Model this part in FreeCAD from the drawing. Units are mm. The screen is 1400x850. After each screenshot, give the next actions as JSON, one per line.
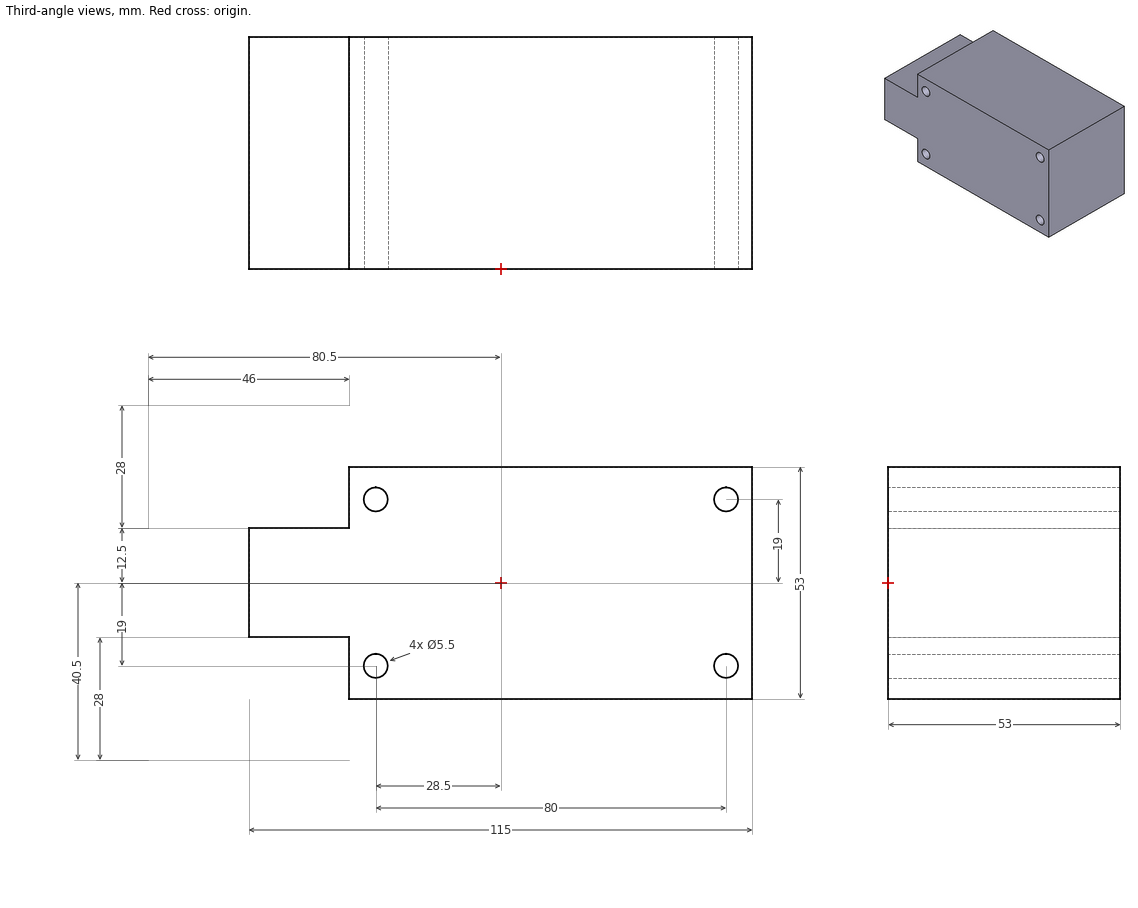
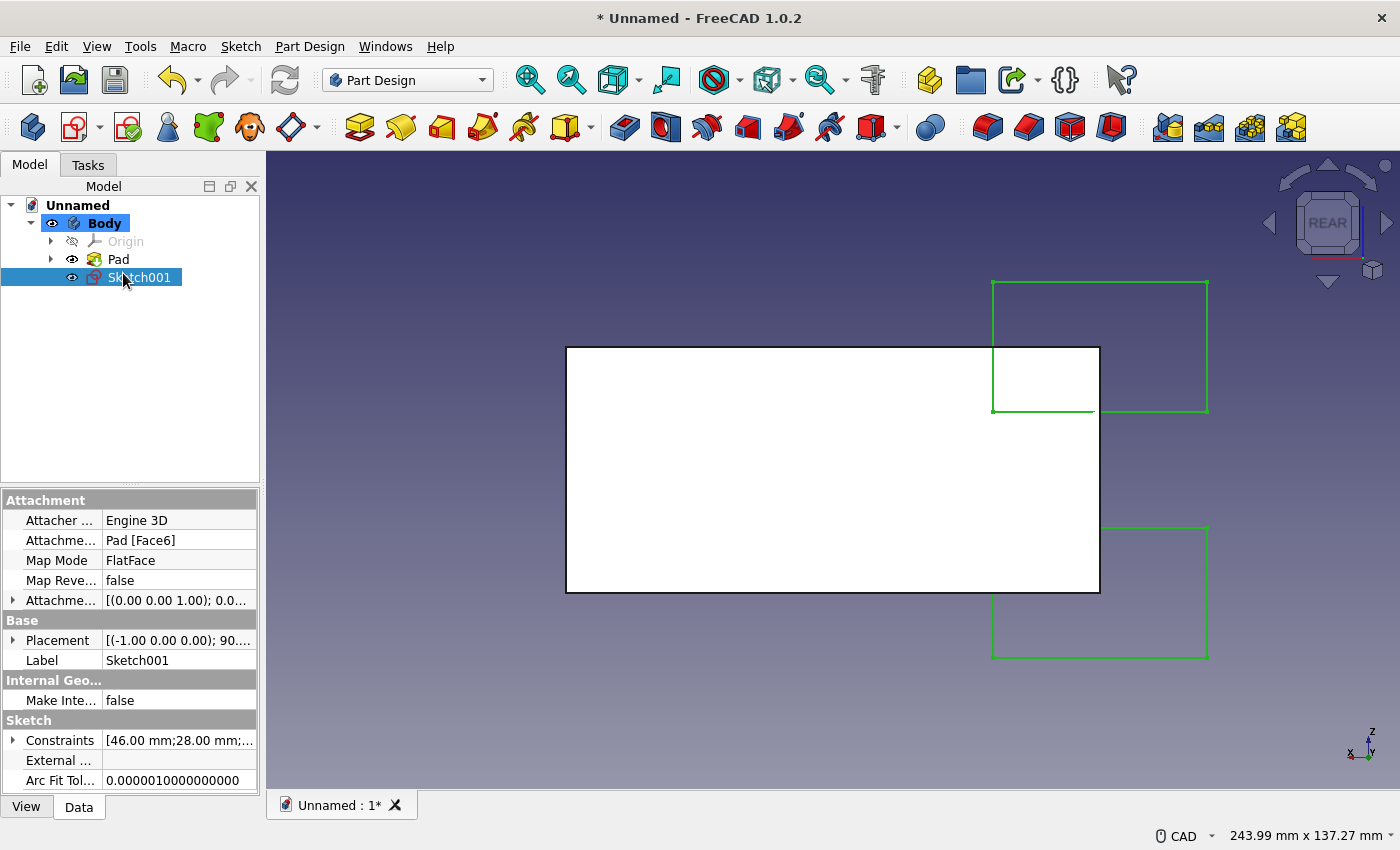
{"action": "left_click", "coordinate": [625, 128]}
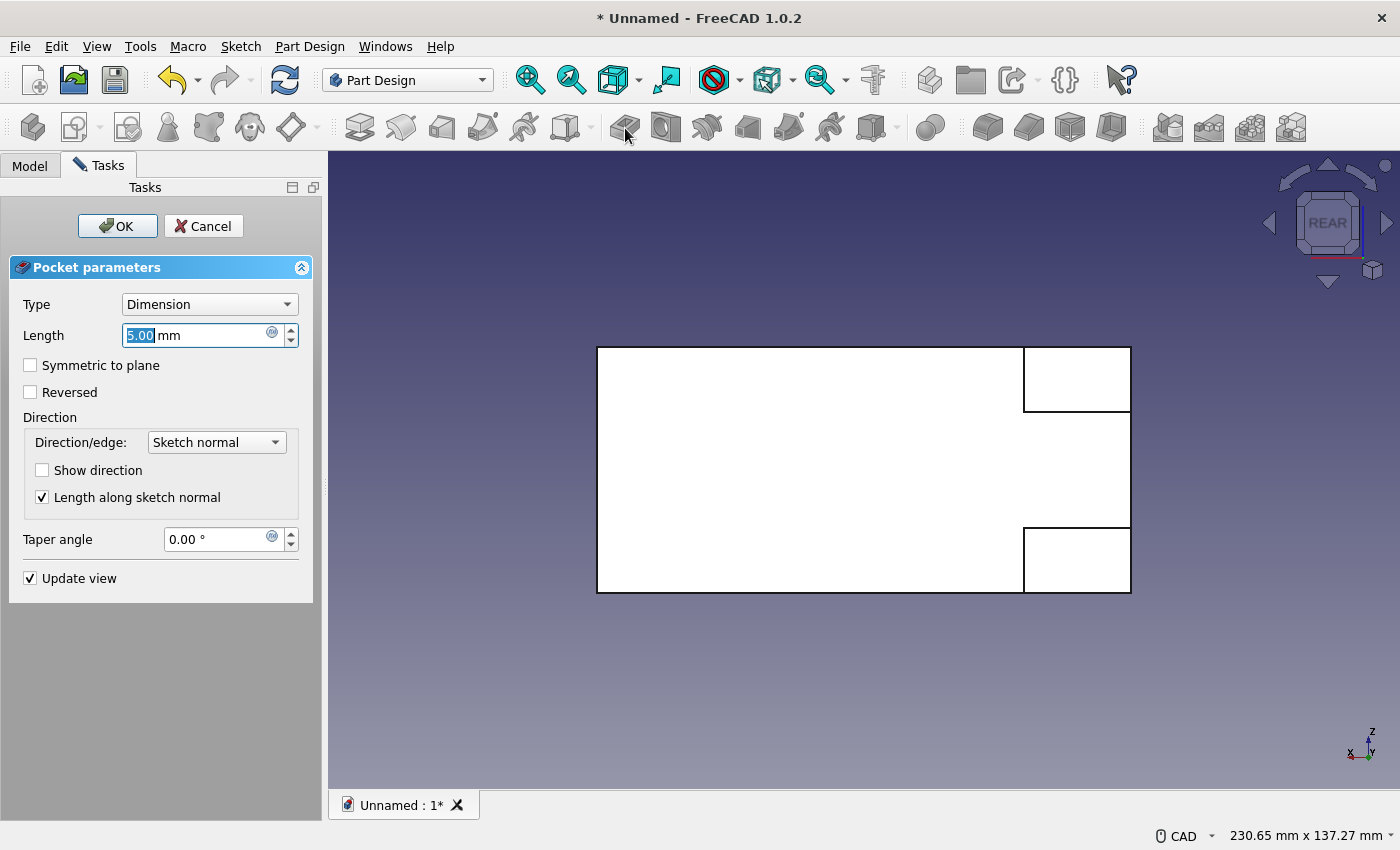
{"action": "left_click", "coordinate": [210, 304]}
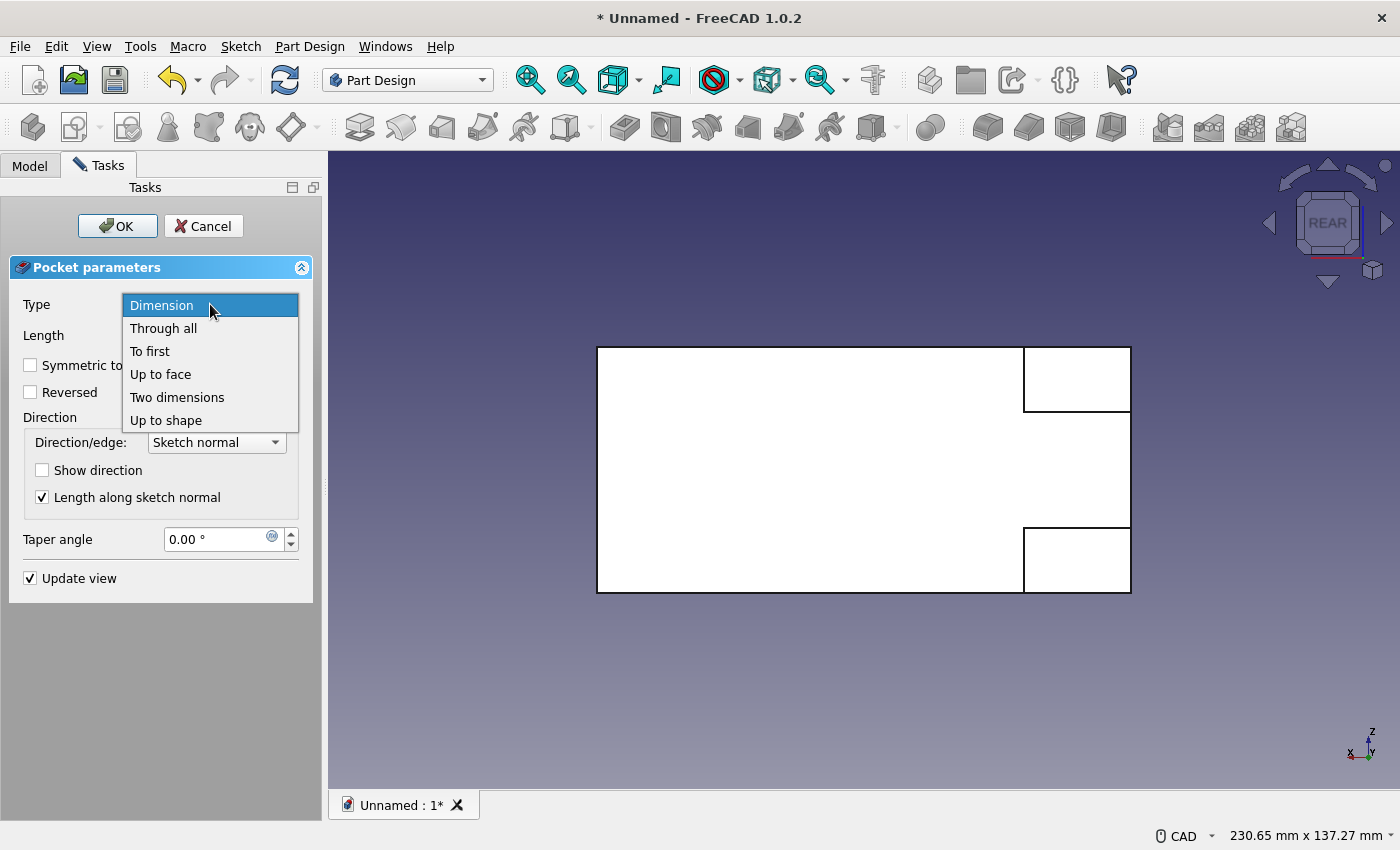
{"action": "left_click", "coordinate": [208, 328]}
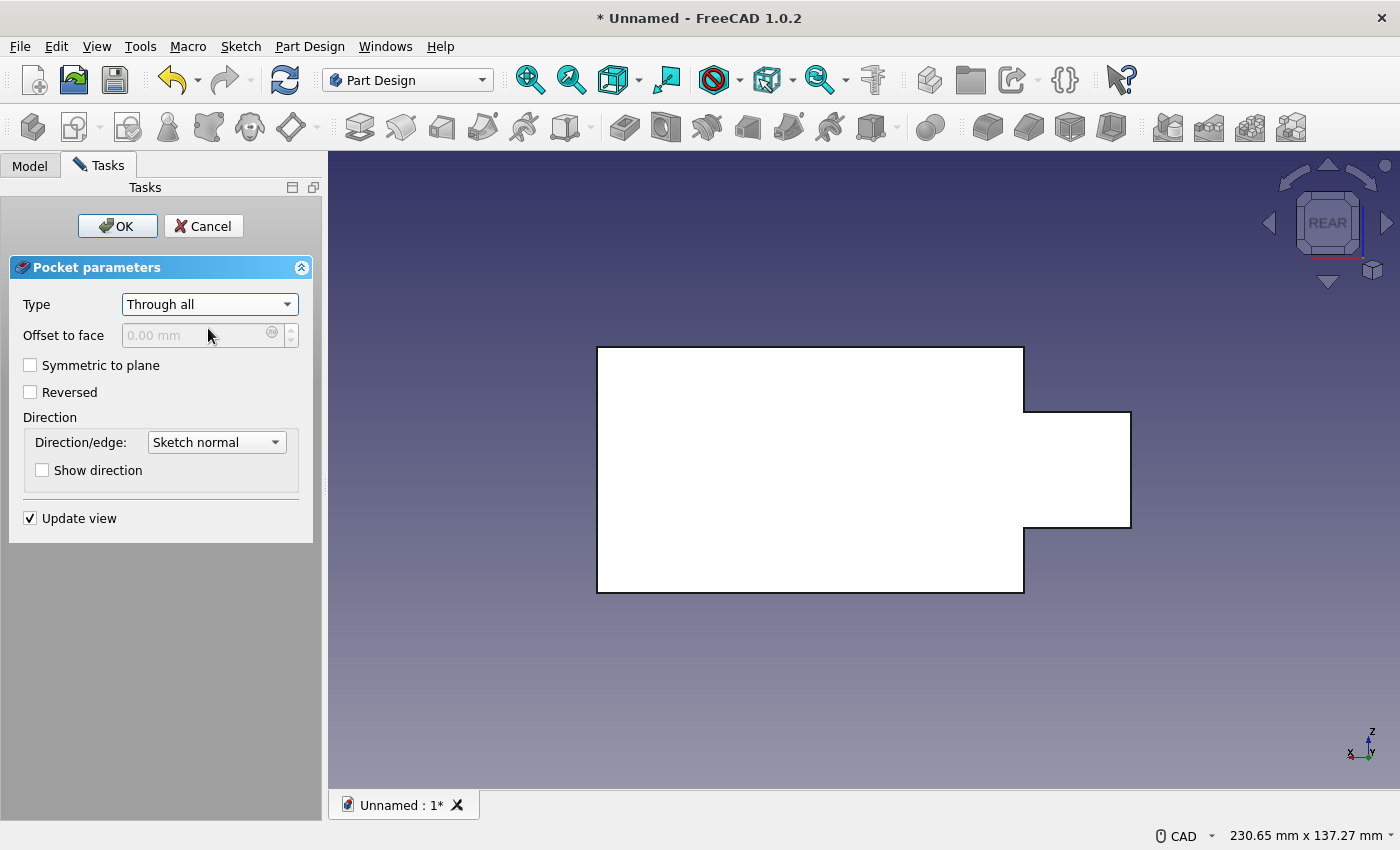
{"action": "left_click", "coordinate": [118, 226]}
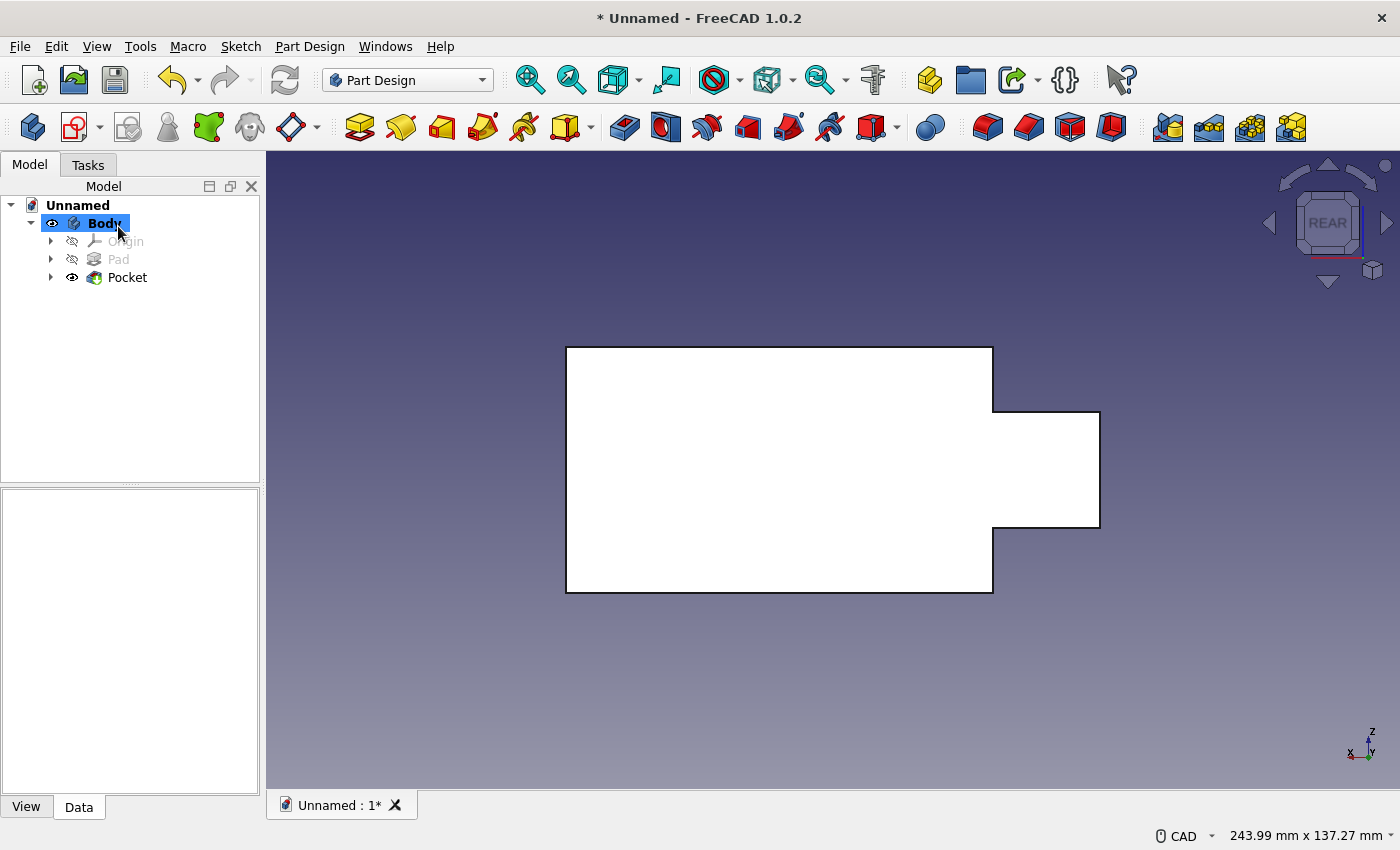
{"action": "left_click", "coordinate": [757, 469]}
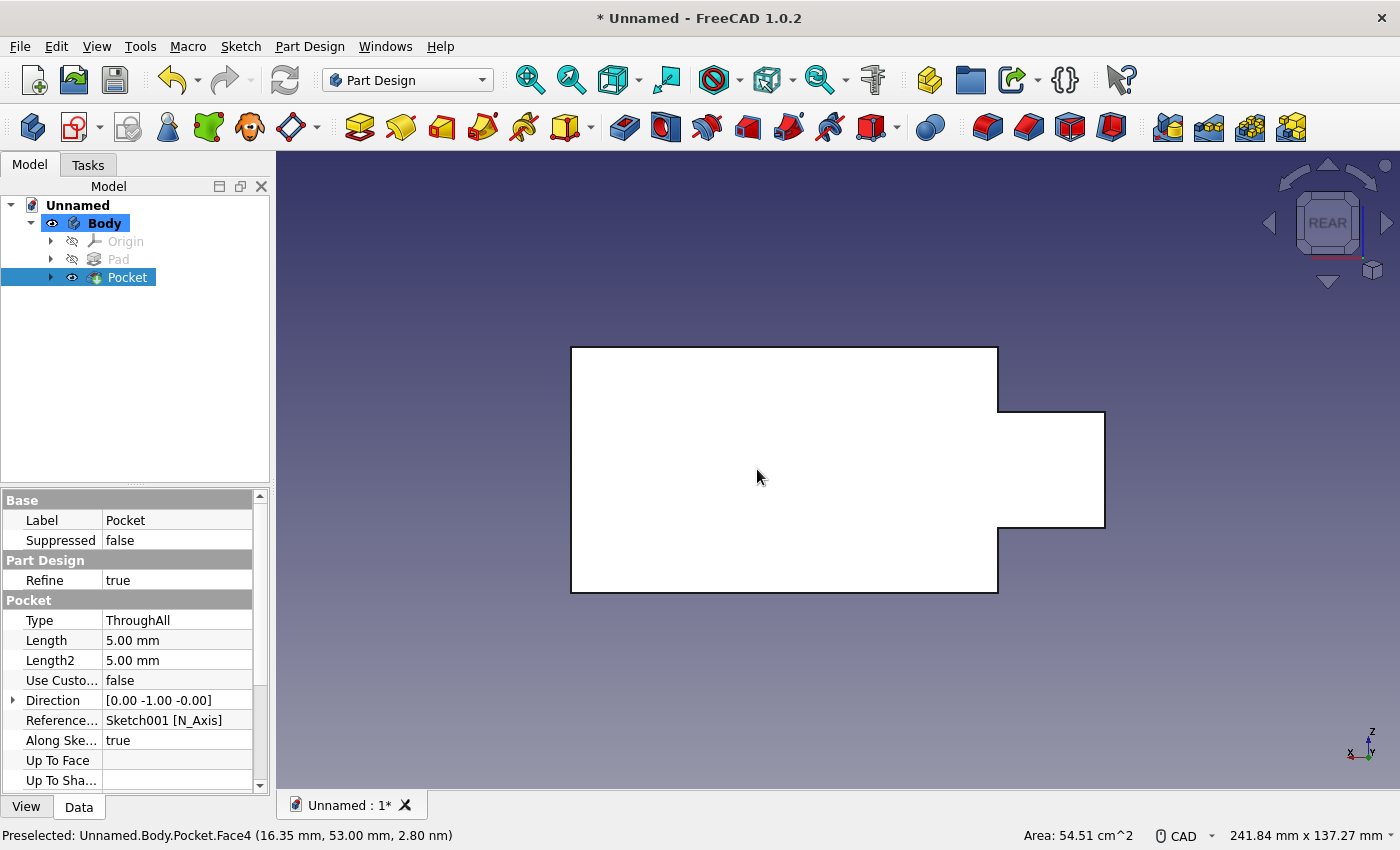
{"action": "left_click", "coordinate": [74, 128]}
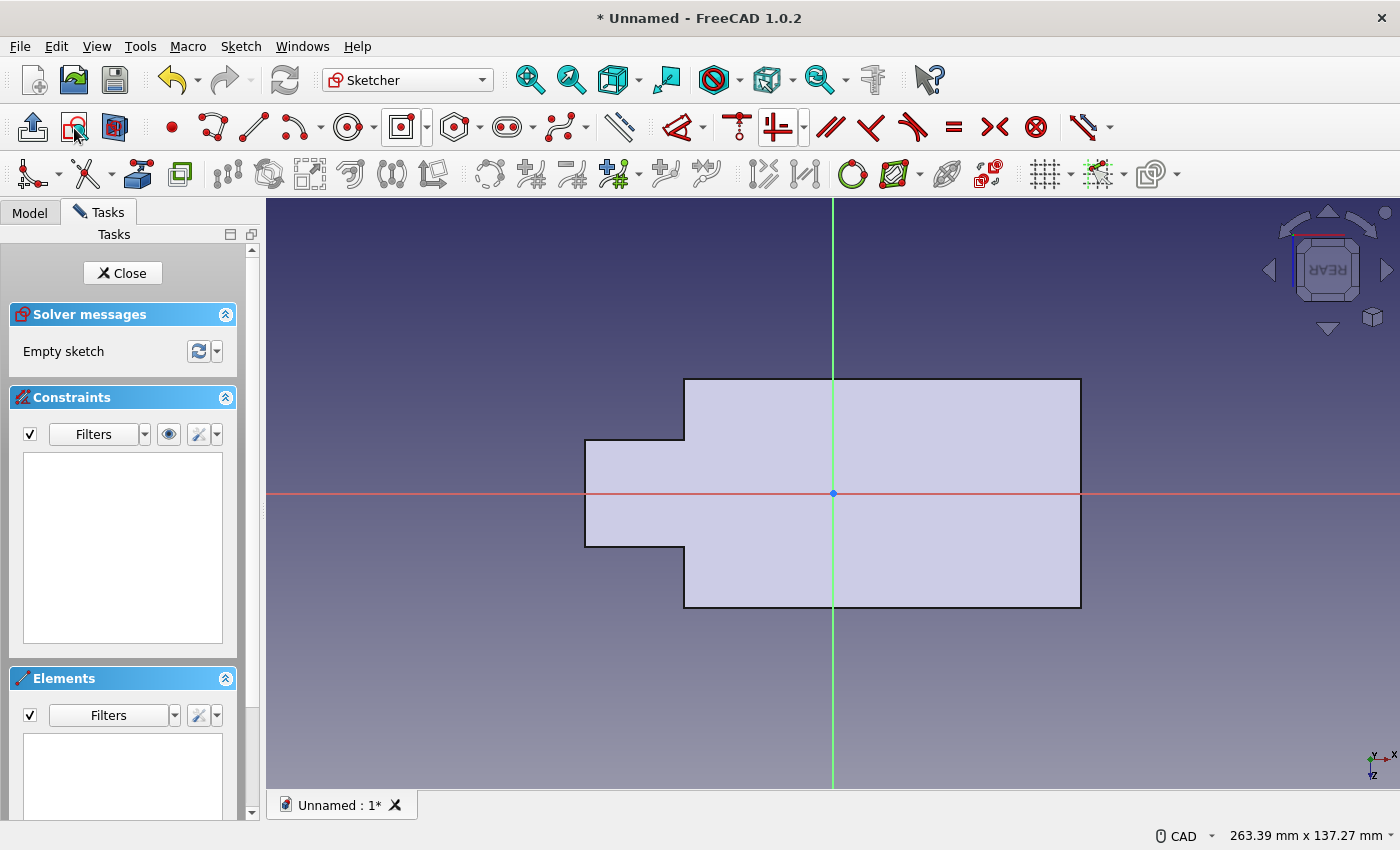
{"action": "scroll", "coordinate": [1026, 493], "scroll_direction": "up", "scroll_amount": 3}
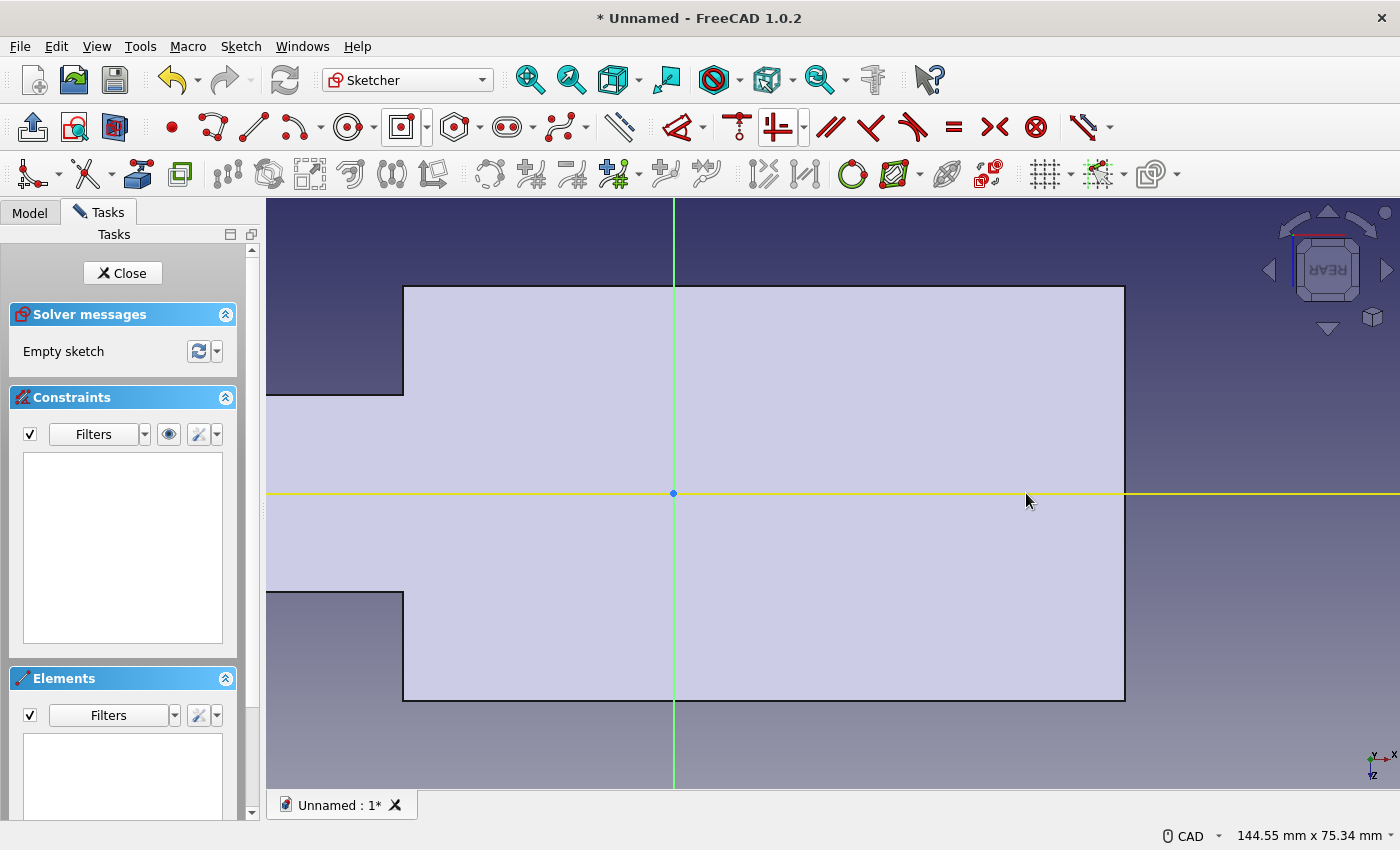
{"action": "left_click", "coordinate": [348, 128]}